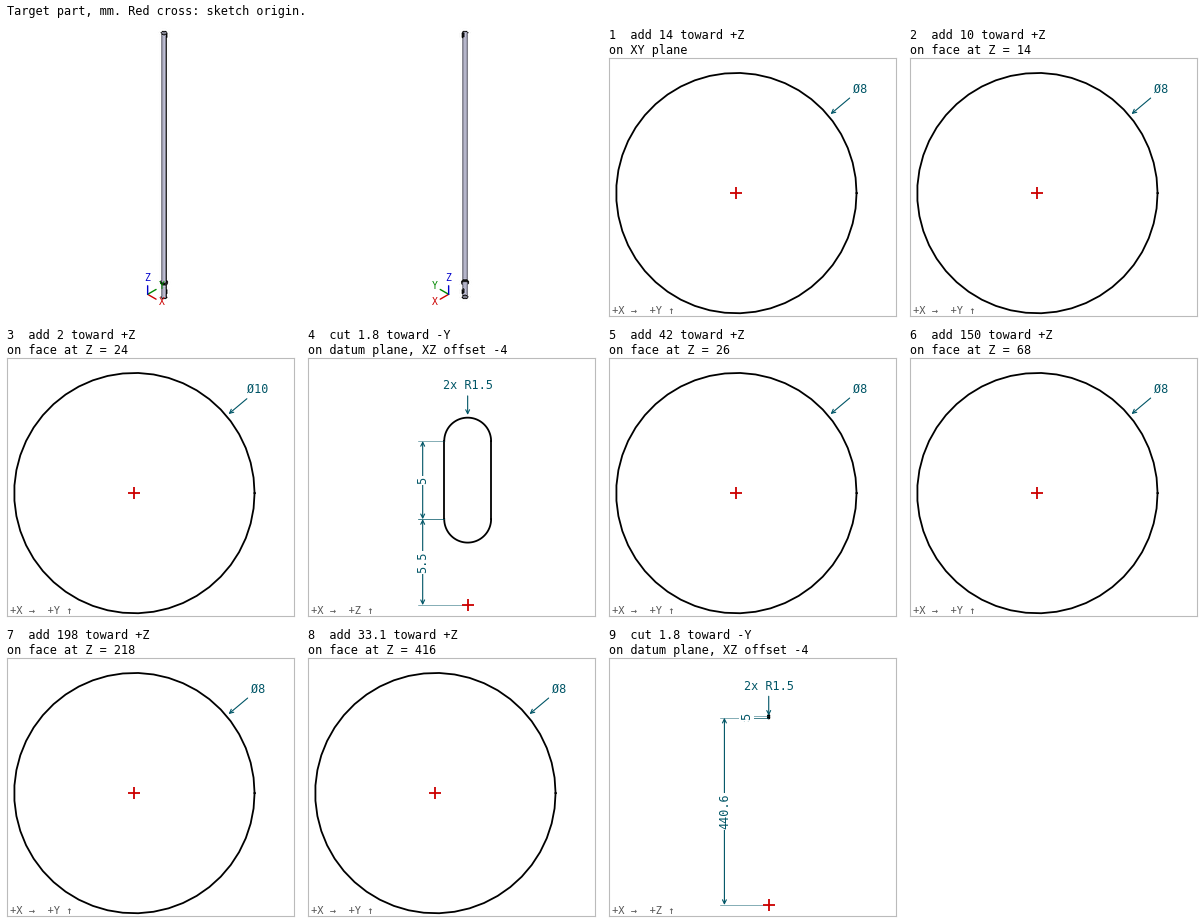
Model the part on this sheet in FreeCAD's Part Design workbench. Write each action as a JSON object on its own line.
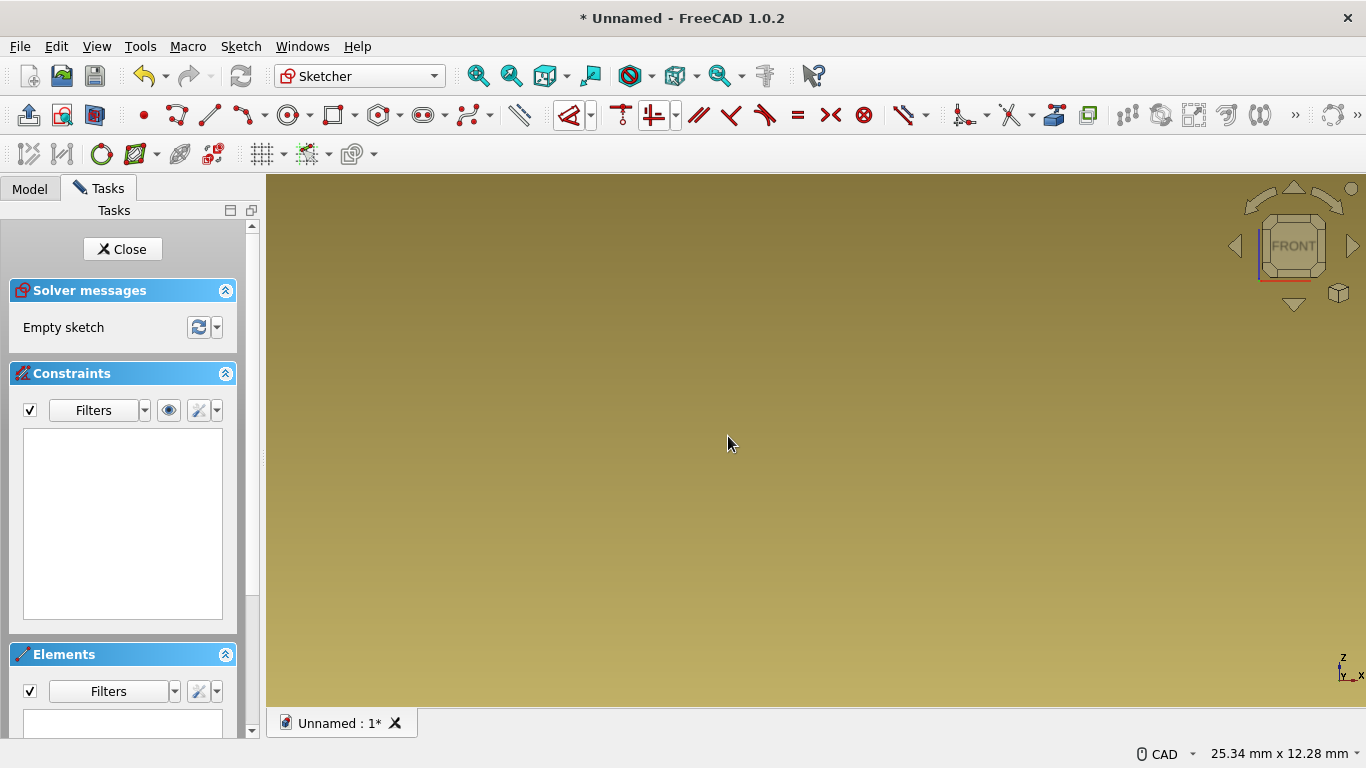
{"action": "left_click", "coordinate": [422, 116]}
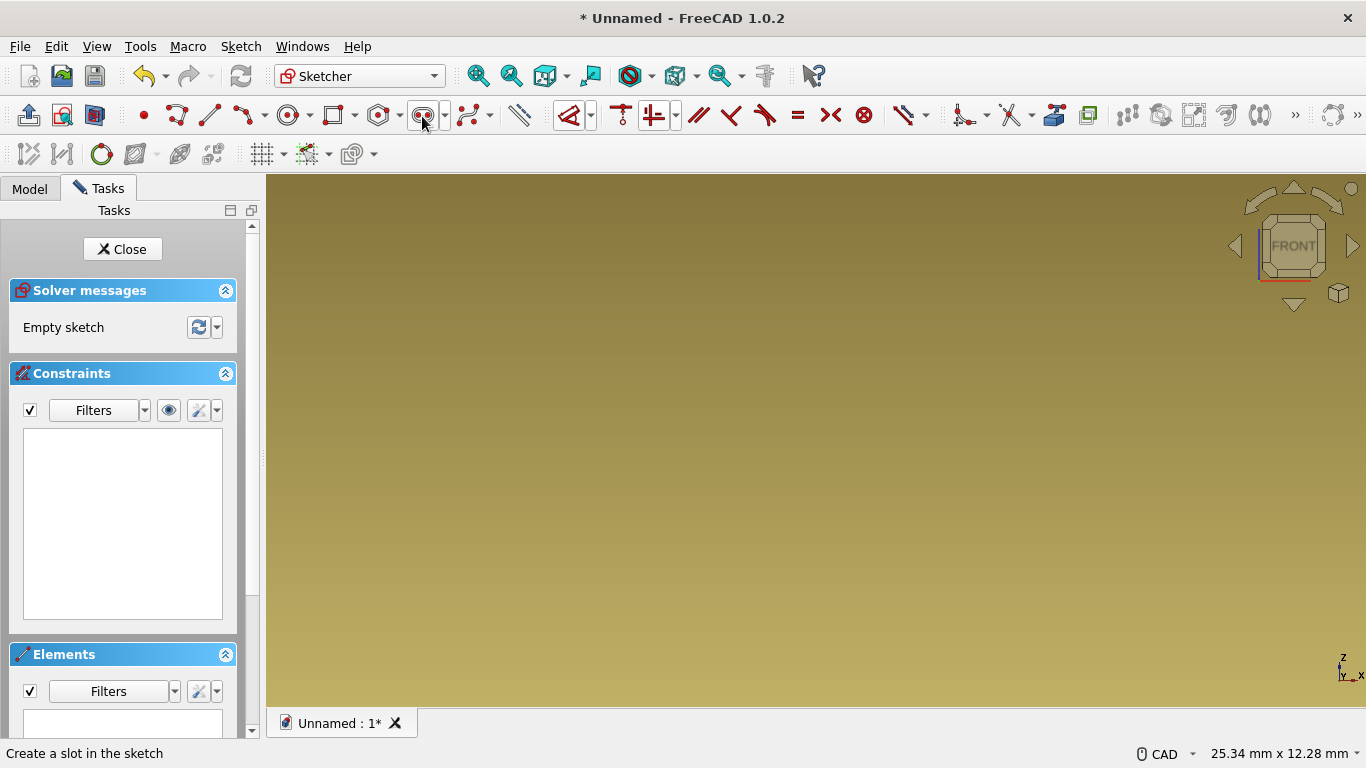
{"action": "left_click", "coordinate": [746, 548]}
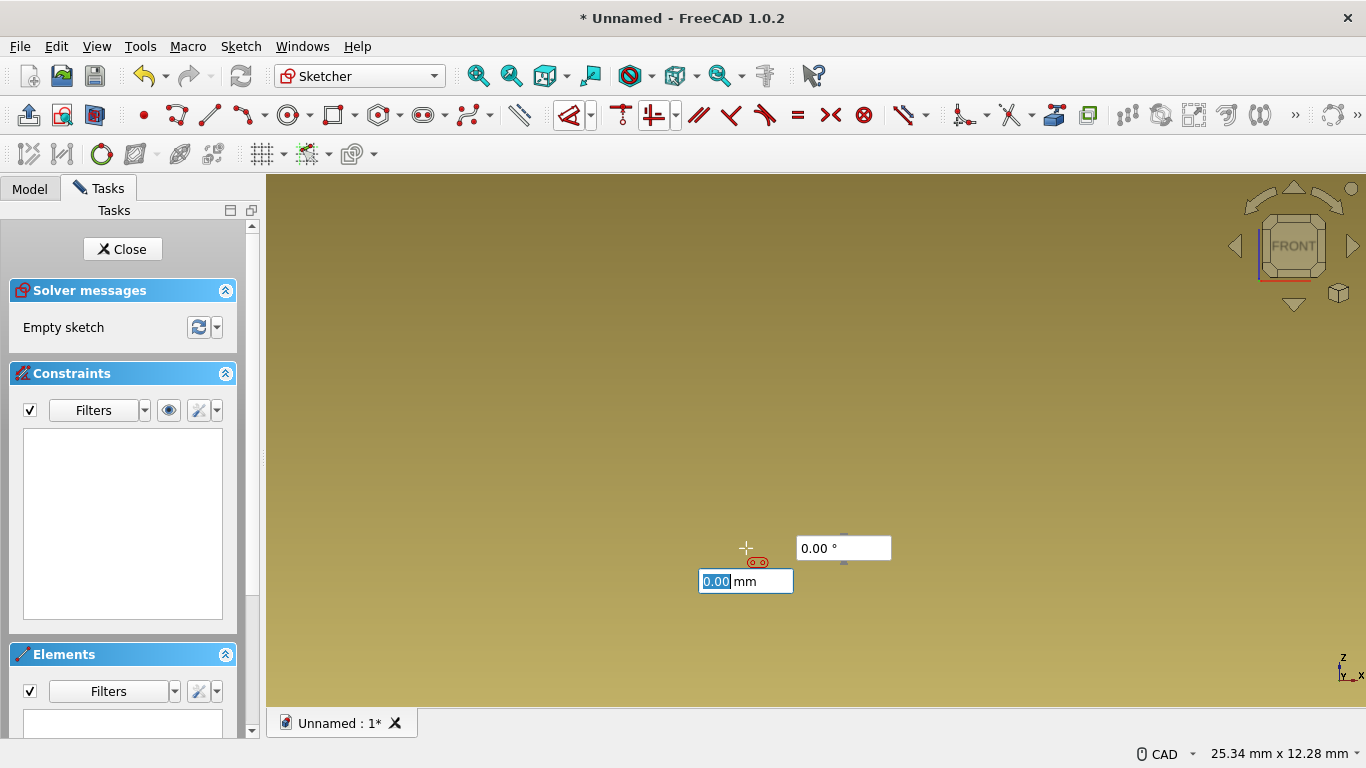
{"action": "left_click", "coordinate": [755, 331]}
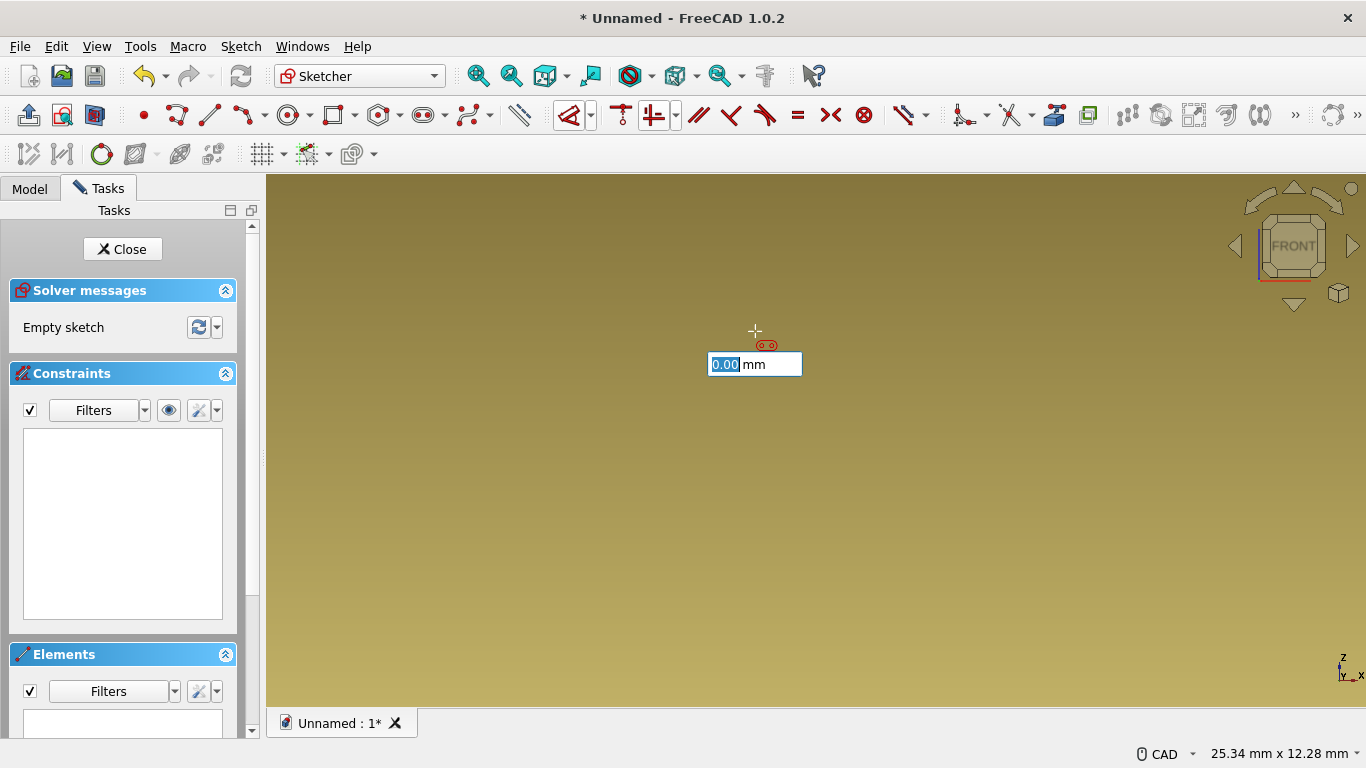
{"action": "left_click", "coordinate": [811, 439]}
{"action": "key", "text": "Escape"}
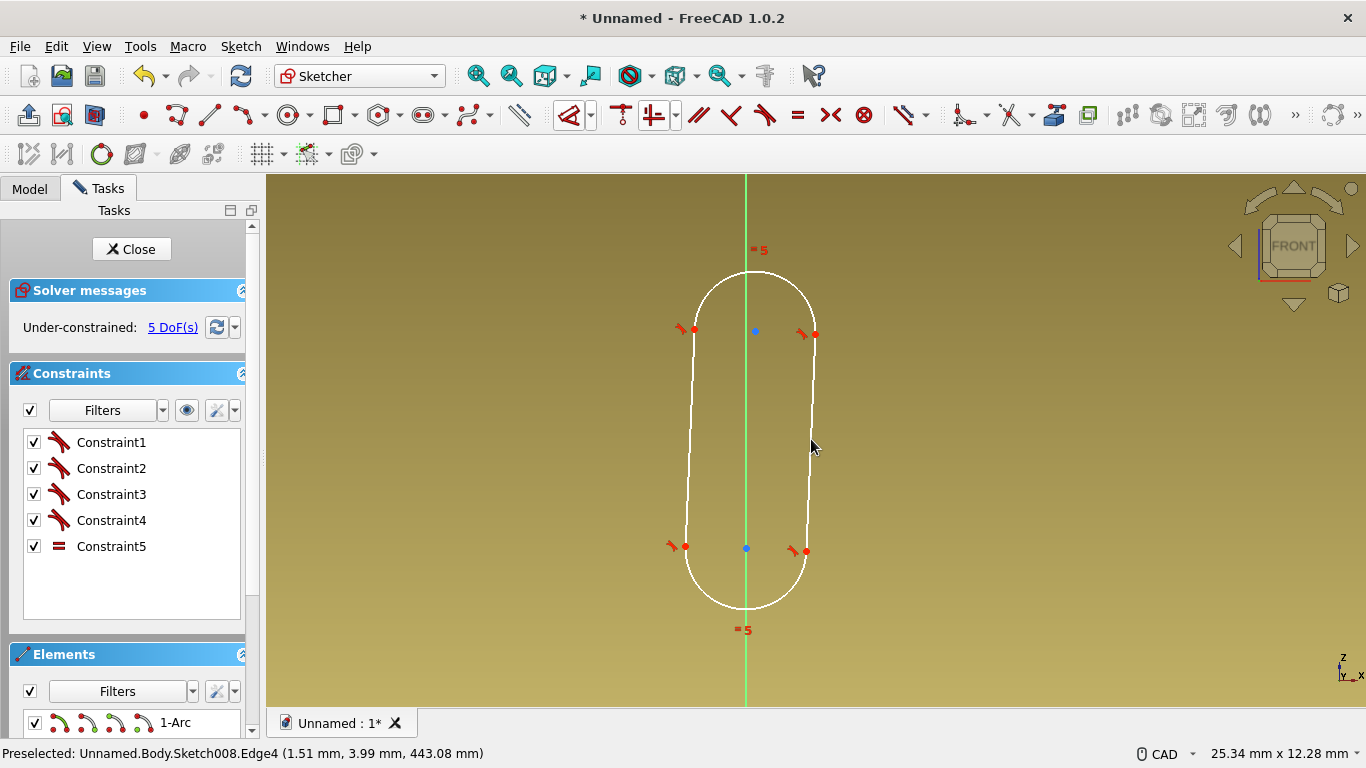
{"action": "left_click", "coordinate": [688, 481]}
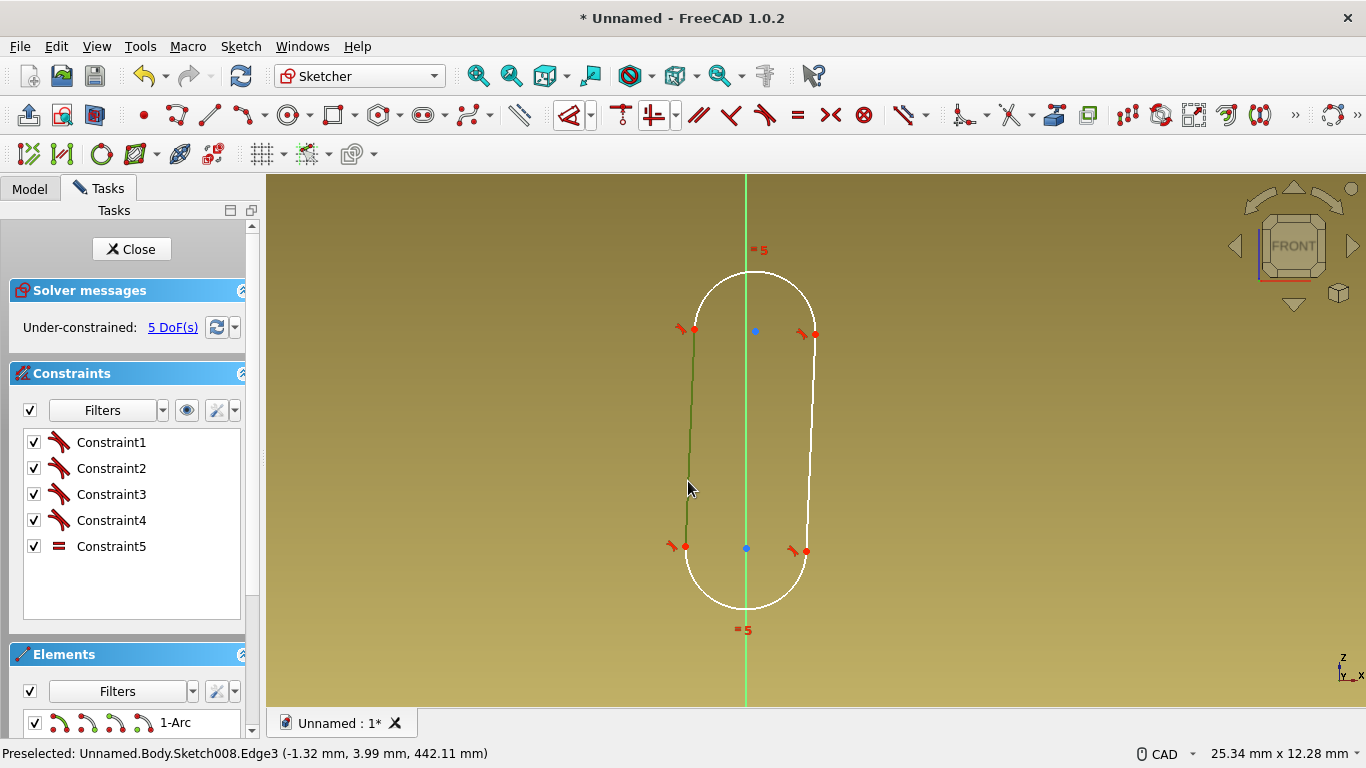
{"action": "key", "text": "v"}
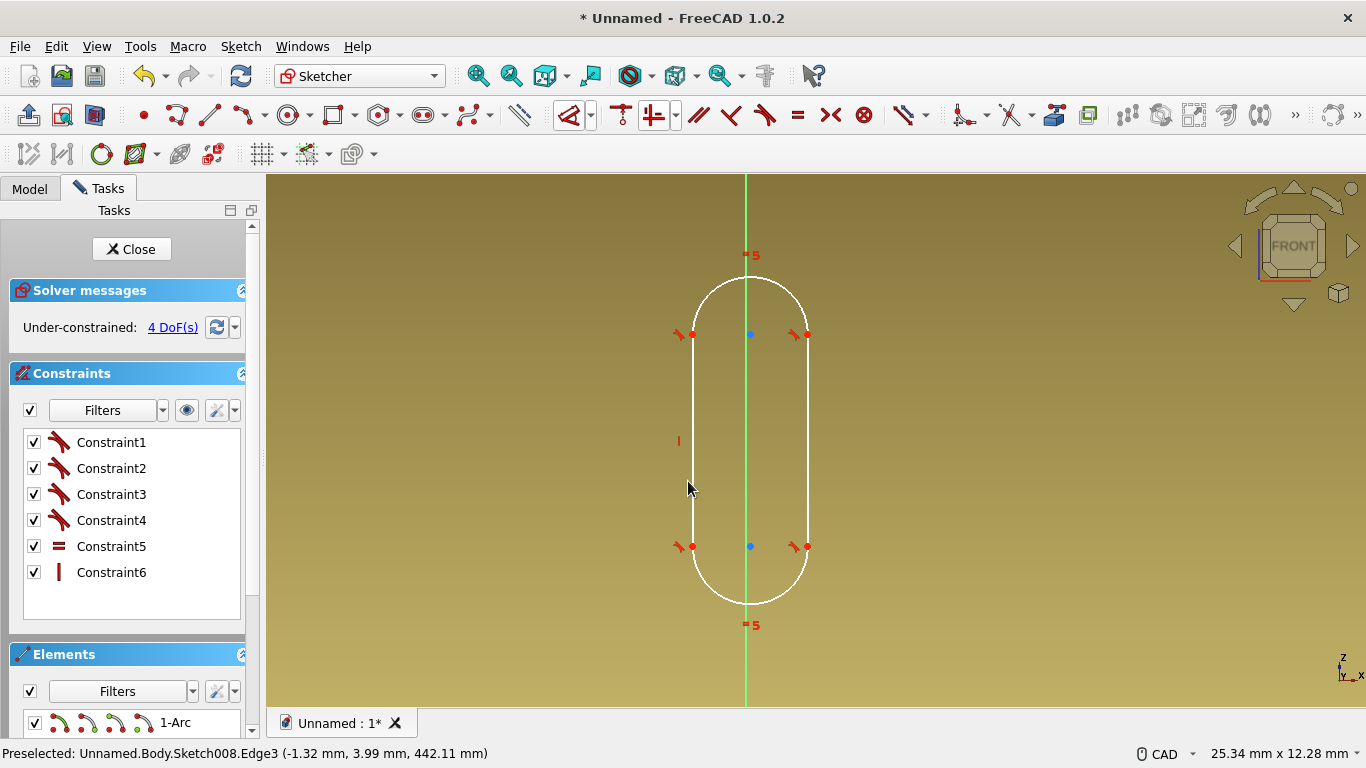
{"action": "left_click", "coordinate": [750, 547]}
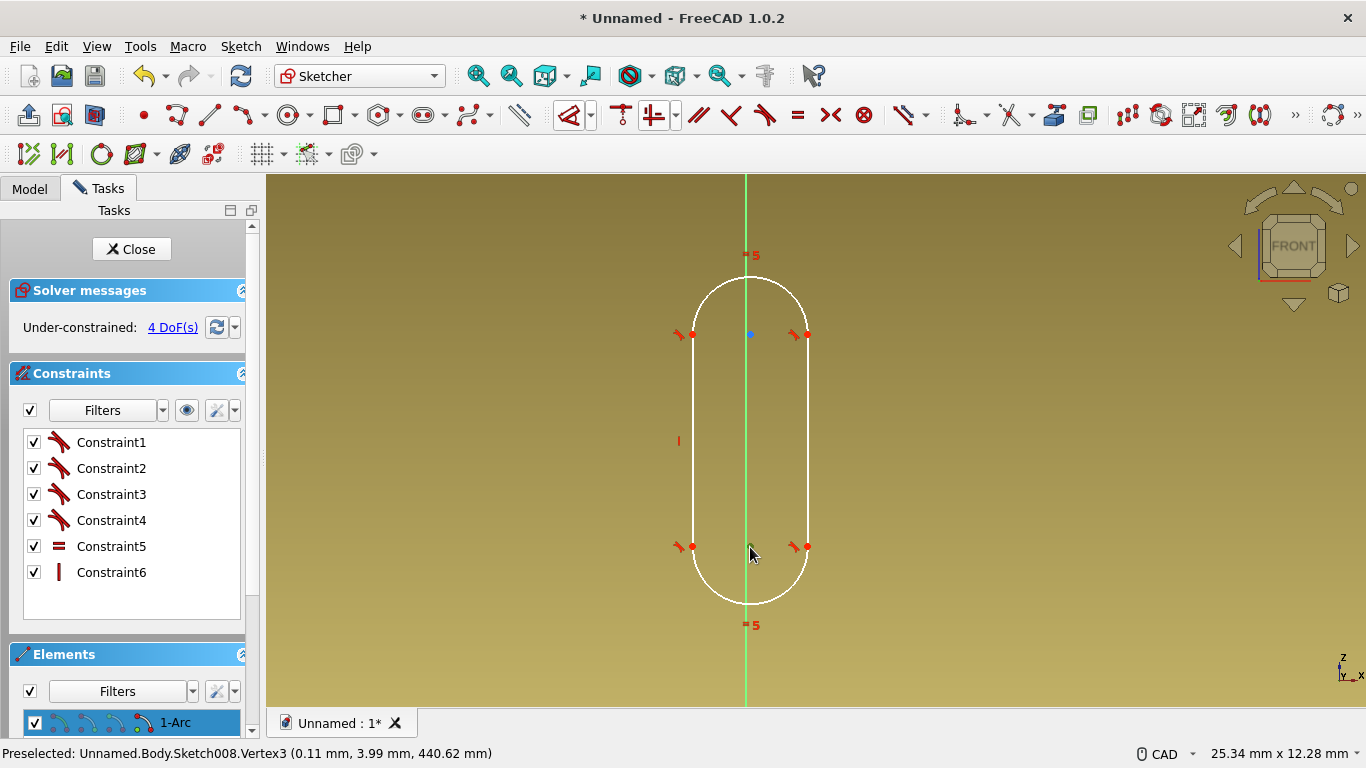
{"action": "left_click", "coordinate": [746, 645]}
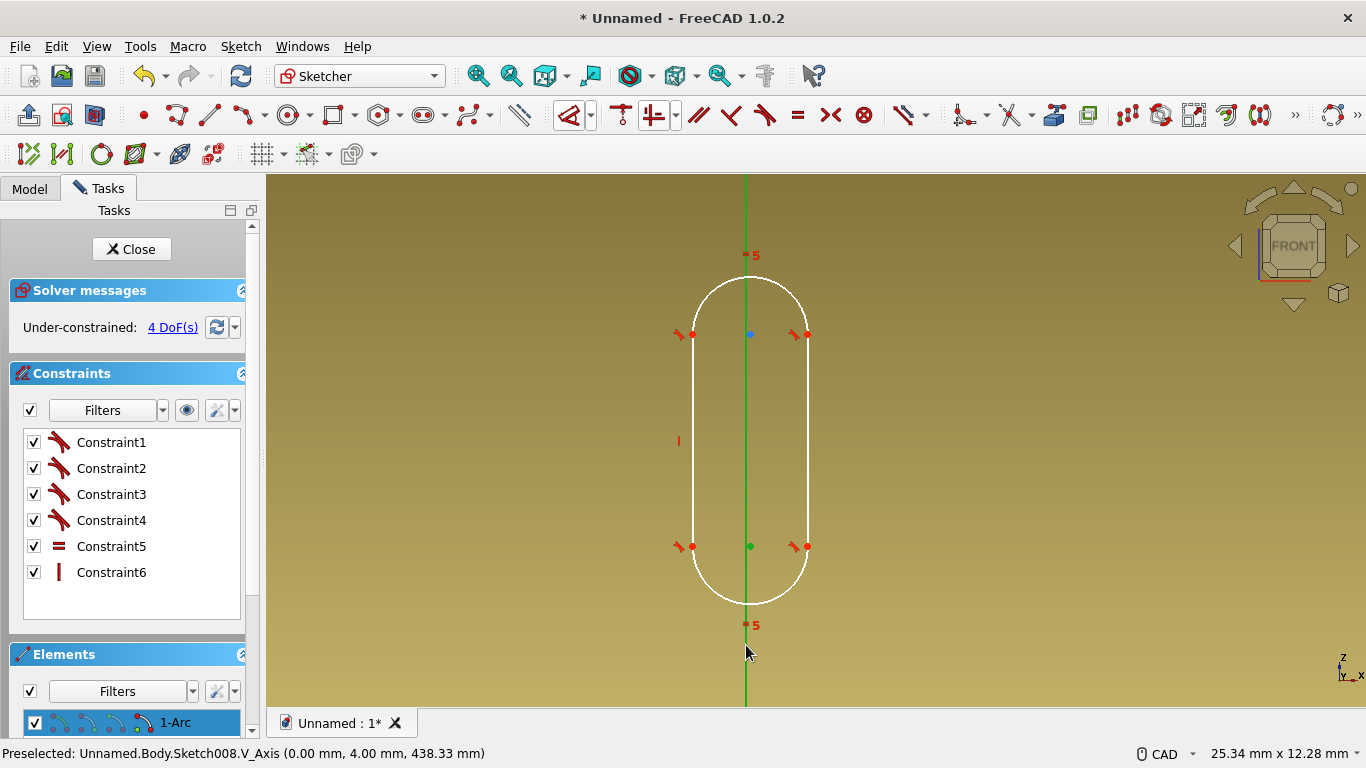
{"action": "left_click", "coordinate": [621, 116]}